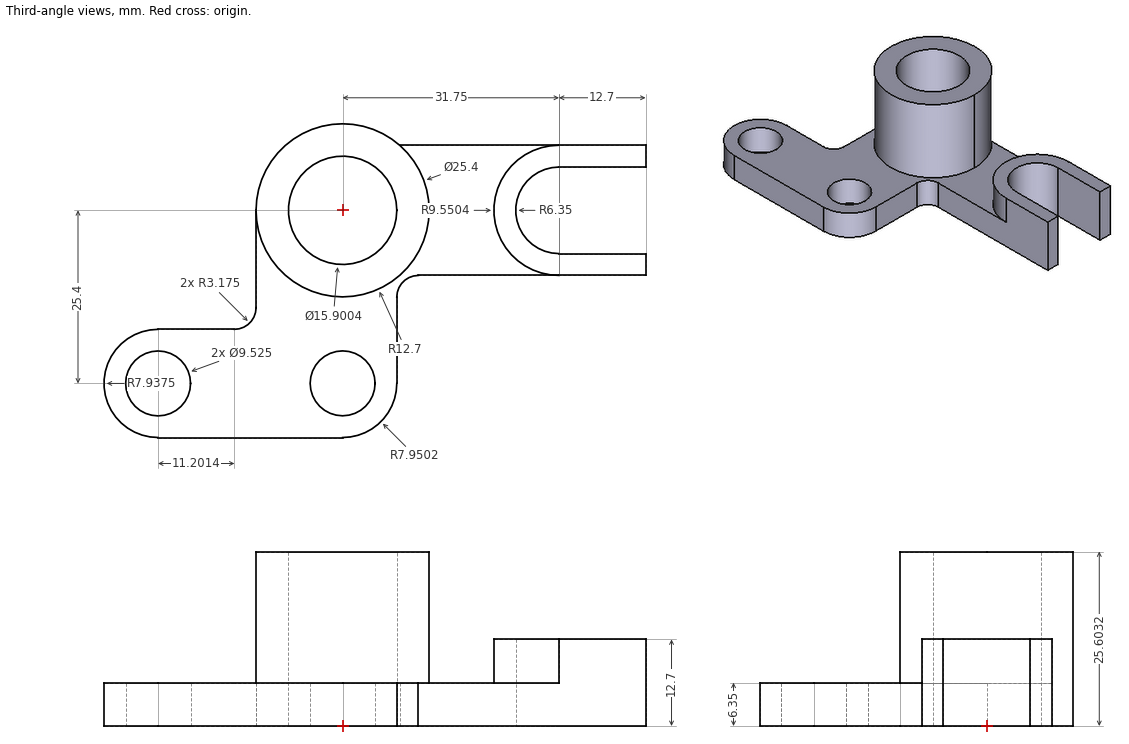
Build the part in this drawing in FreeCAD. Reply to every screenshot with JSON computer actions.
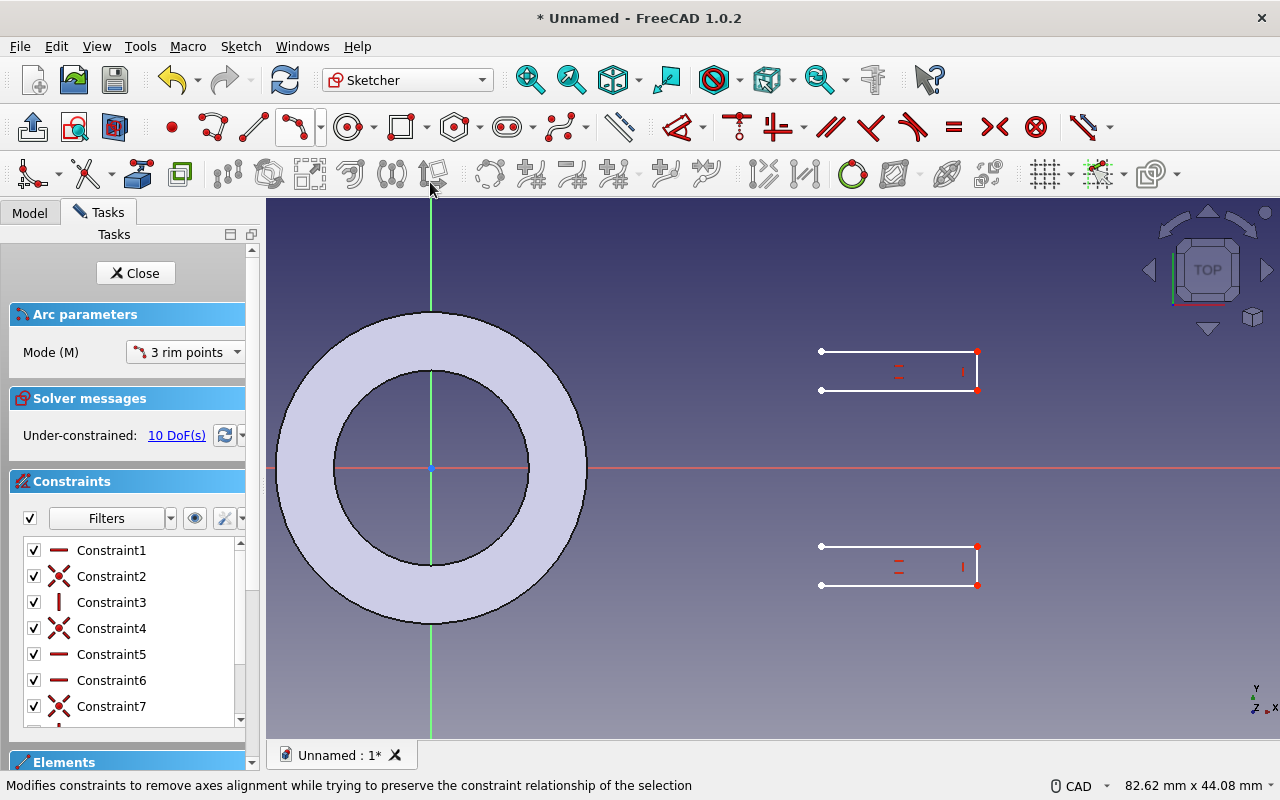
{"action": "left_click", "coordinate": [821, 547]}
{"action": "left_click", "coordinate": [821, 391]}
{"action": "left_click", "coordinate": [747, 444]}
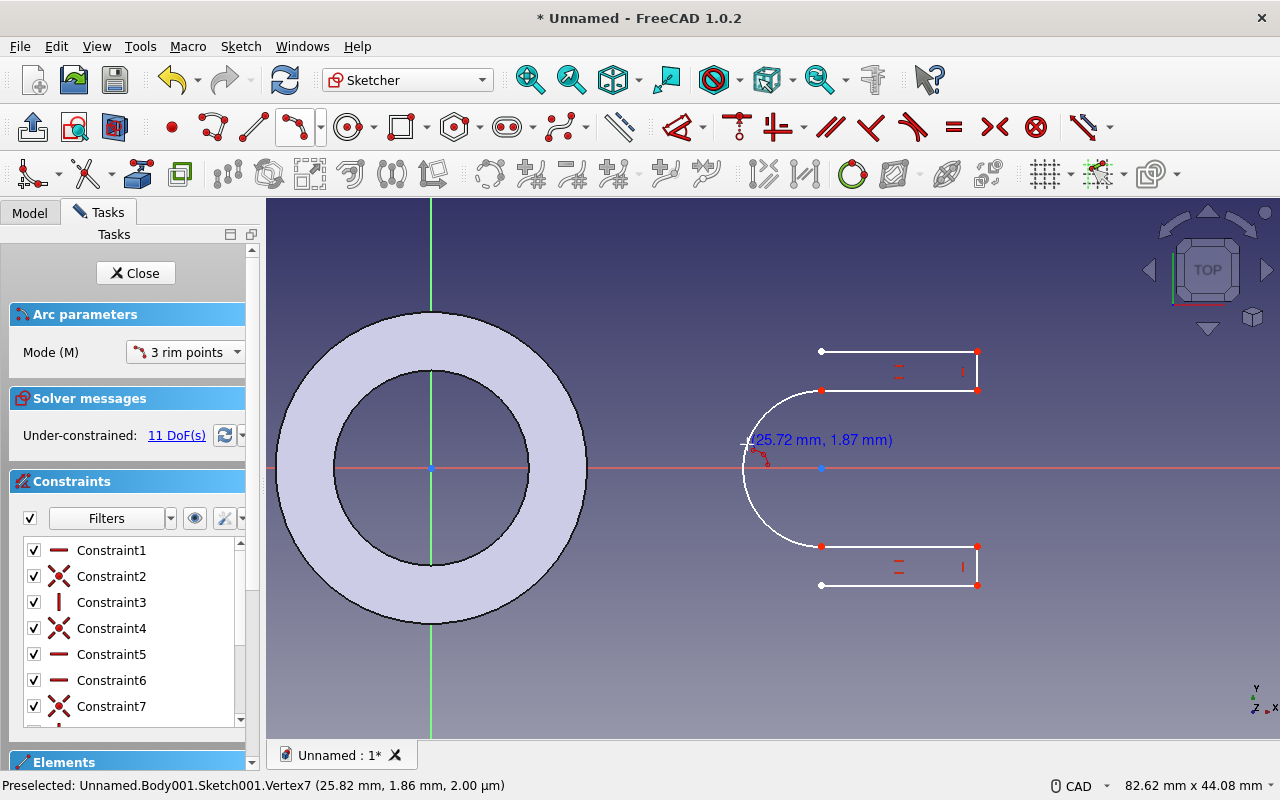
{"action": "left_click", "coordinate": [821, 352]}
{"action": "left_click", "coordinate": [821, 586]}
{"action": "left_click", "coordinate": [710, 432]}
{"action": "key", "text": "Escape"}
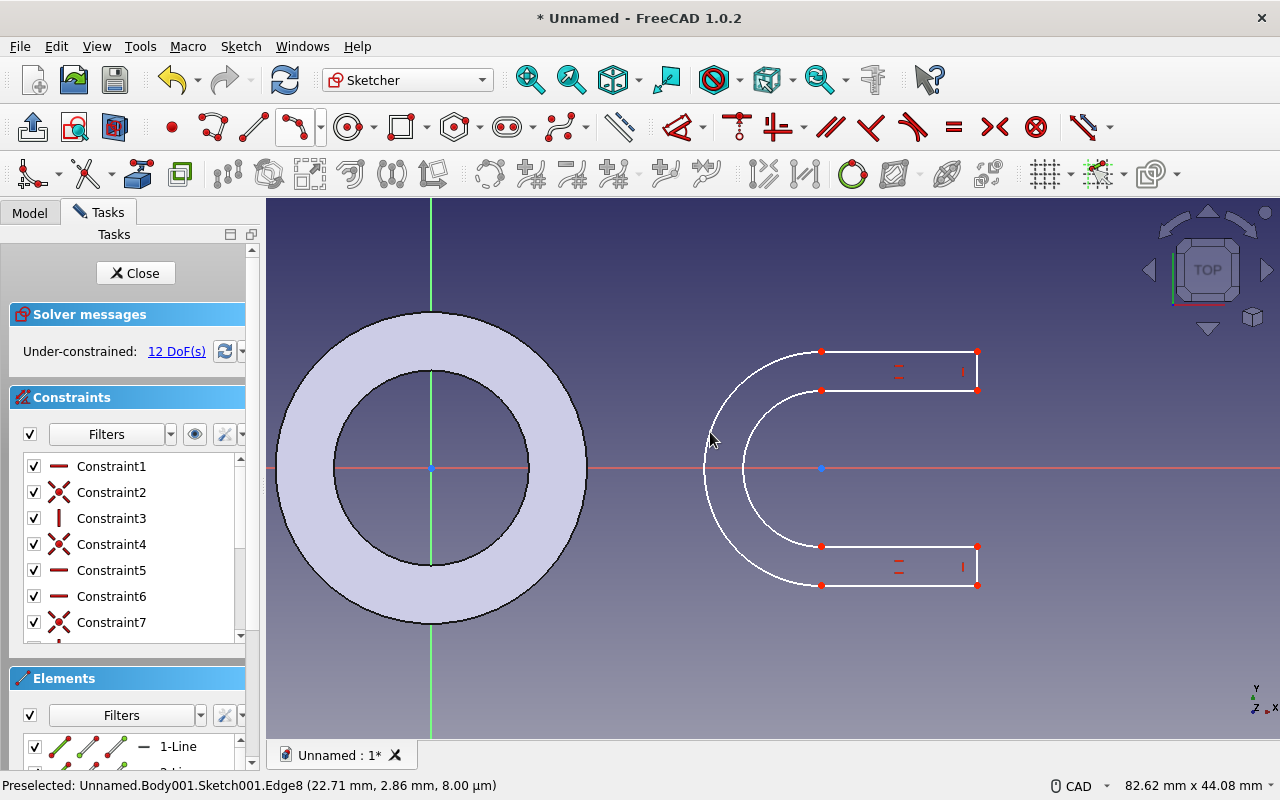
{"action": "left_click", "coordinate": [868, 586]}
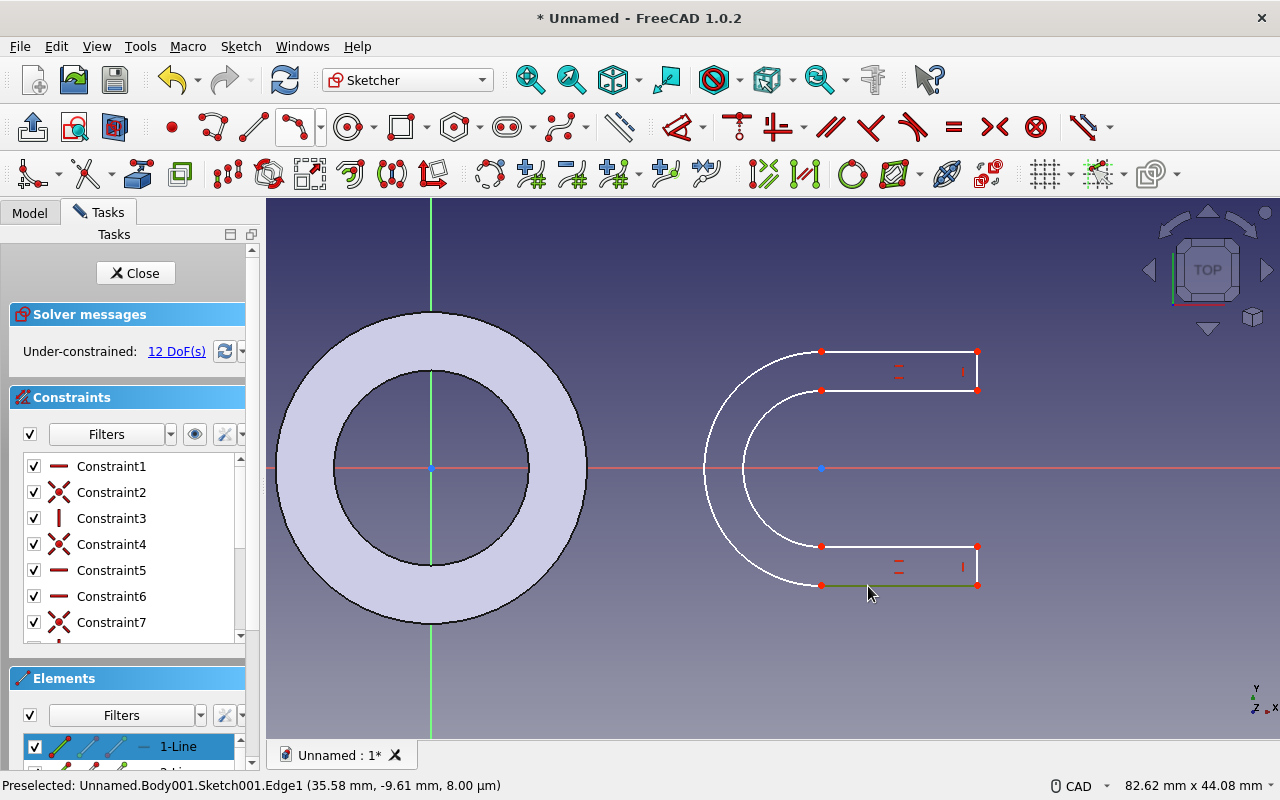
{"action": "left_click", "coordinate": [727, 400]}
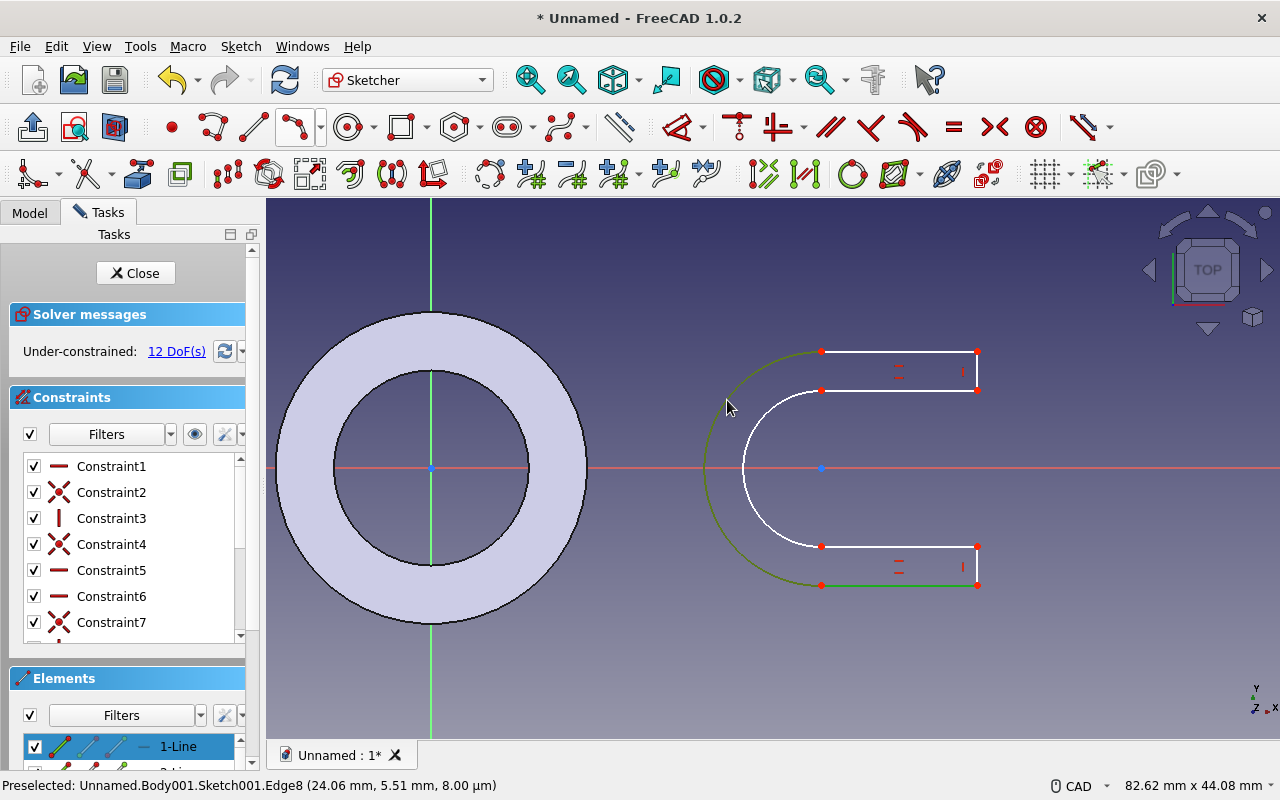
{"action": "left_click", "coordinate": [913, 128]}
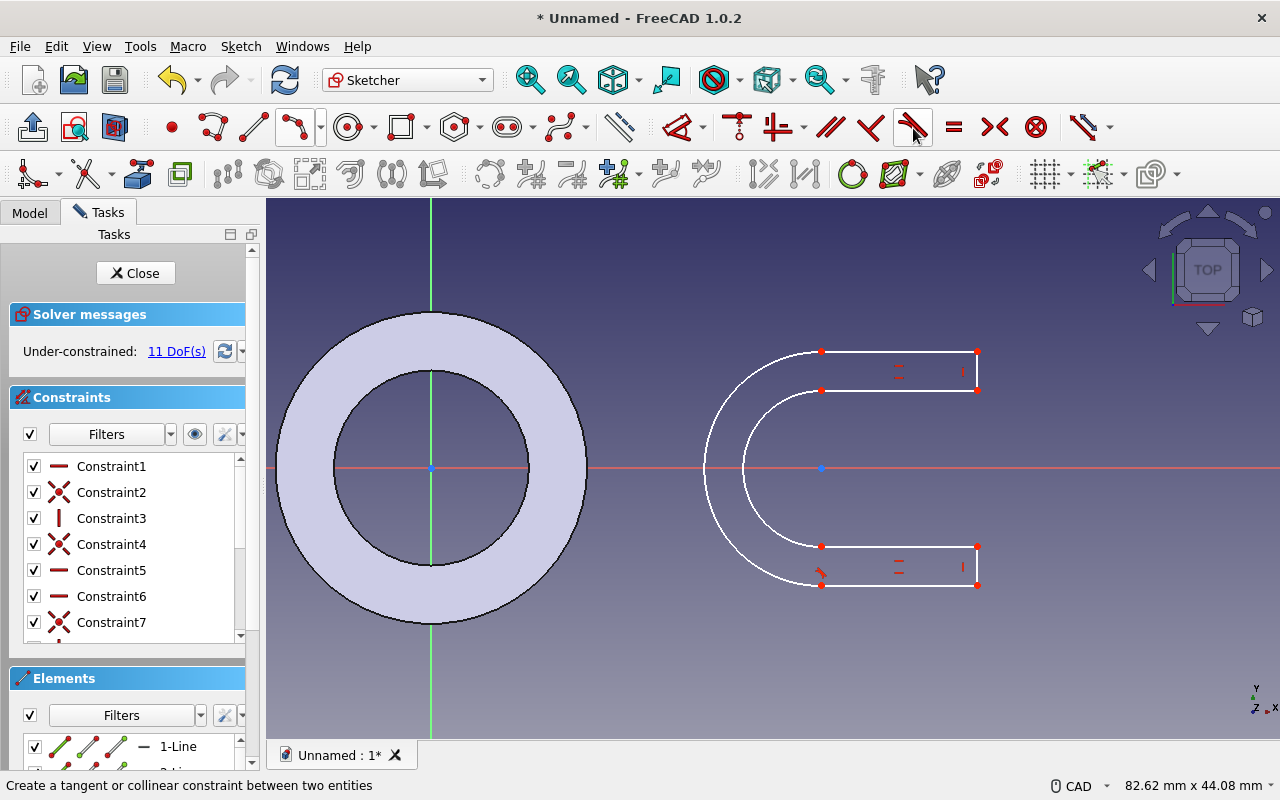
{"action": "left_click", "coordinate": [930, 547]}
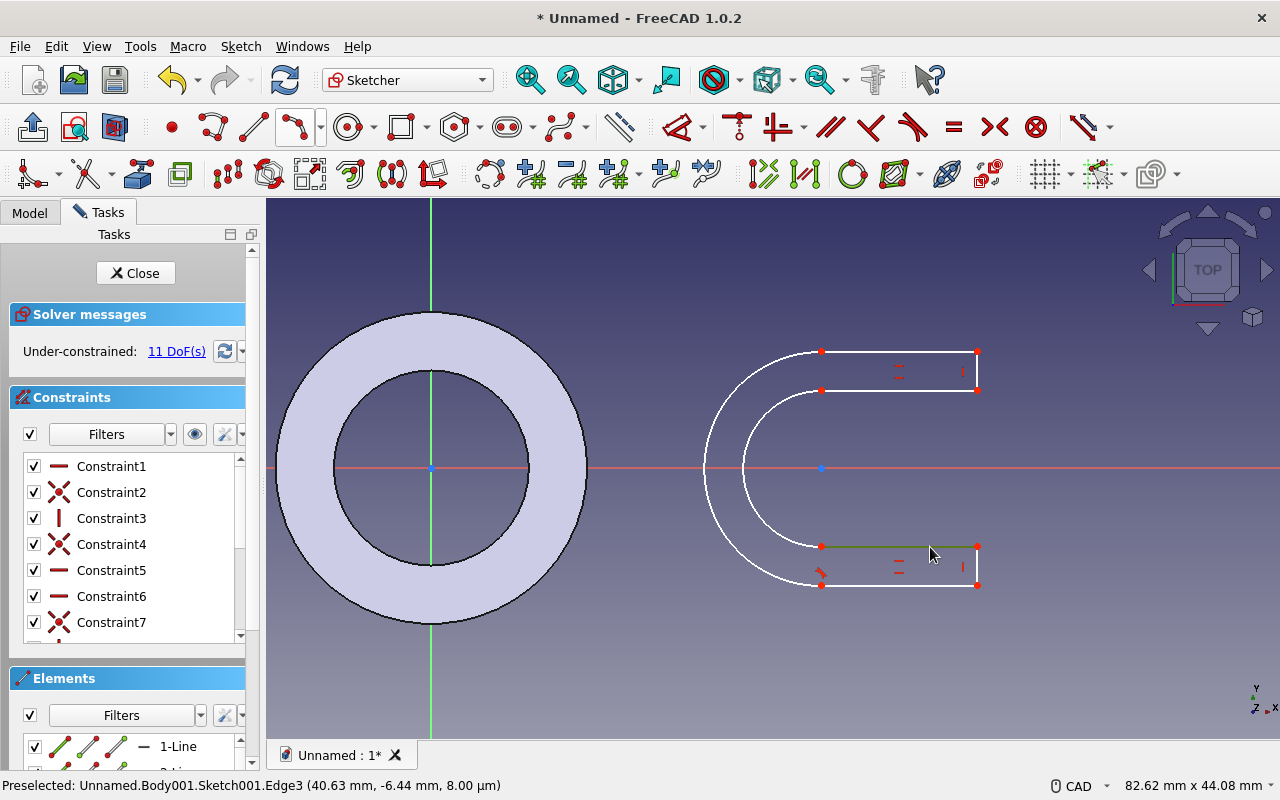
{"action": "left_click", "coordinate": [758, 423]}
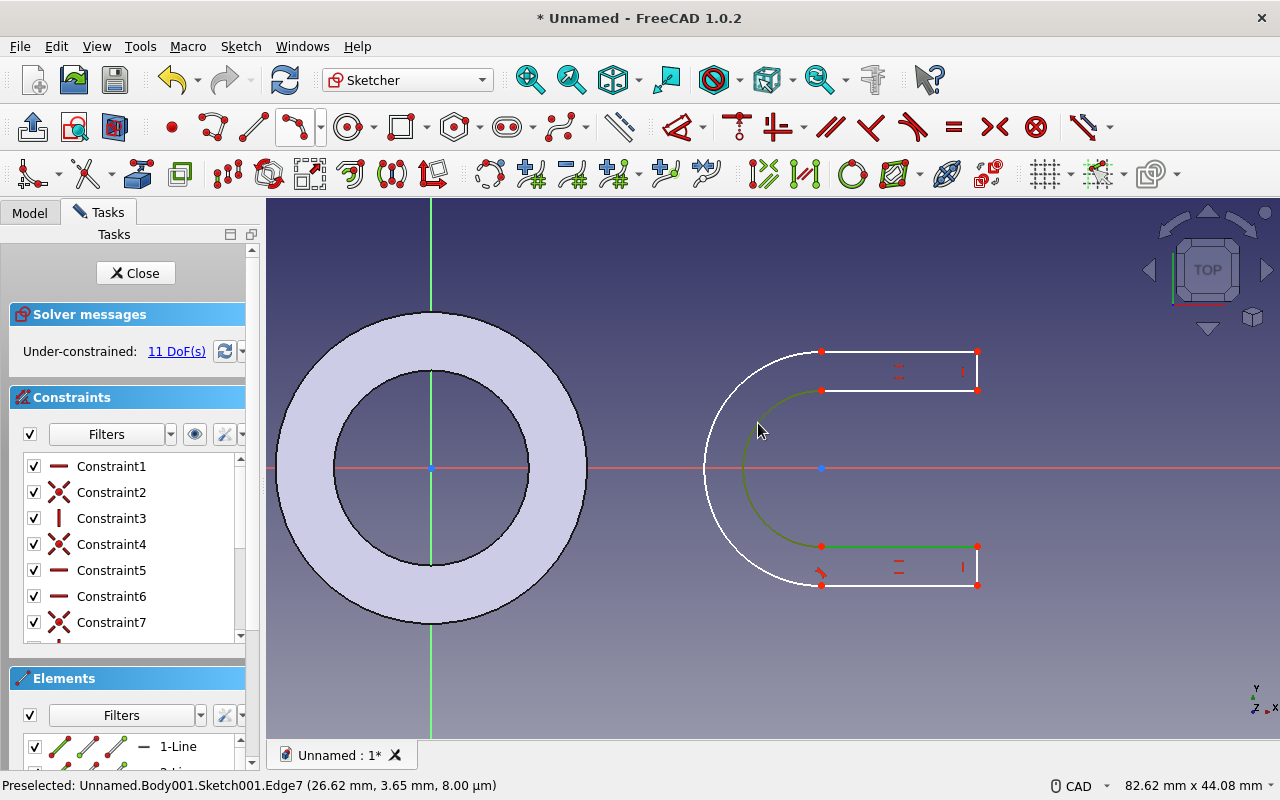
{"action": "key", "text": "t"}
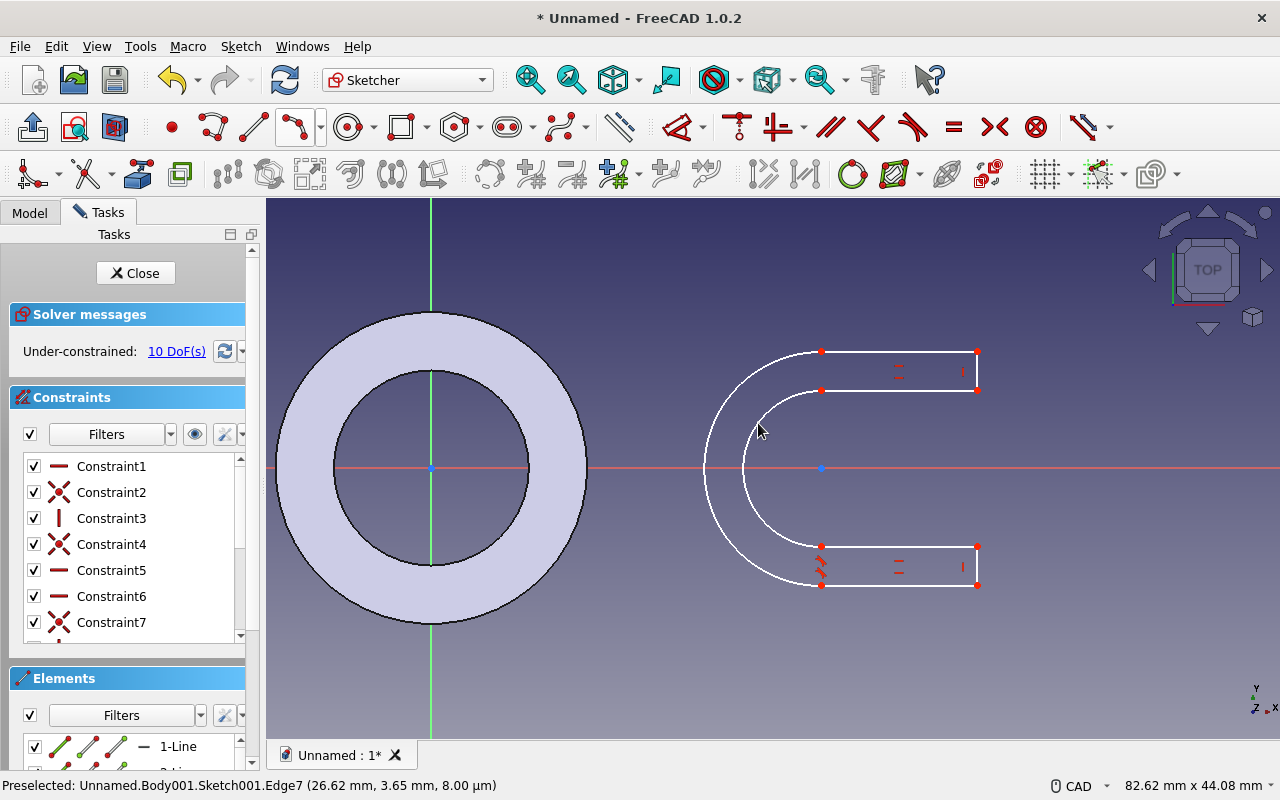
{"action": "left_click", "coordinate": [868, 391]}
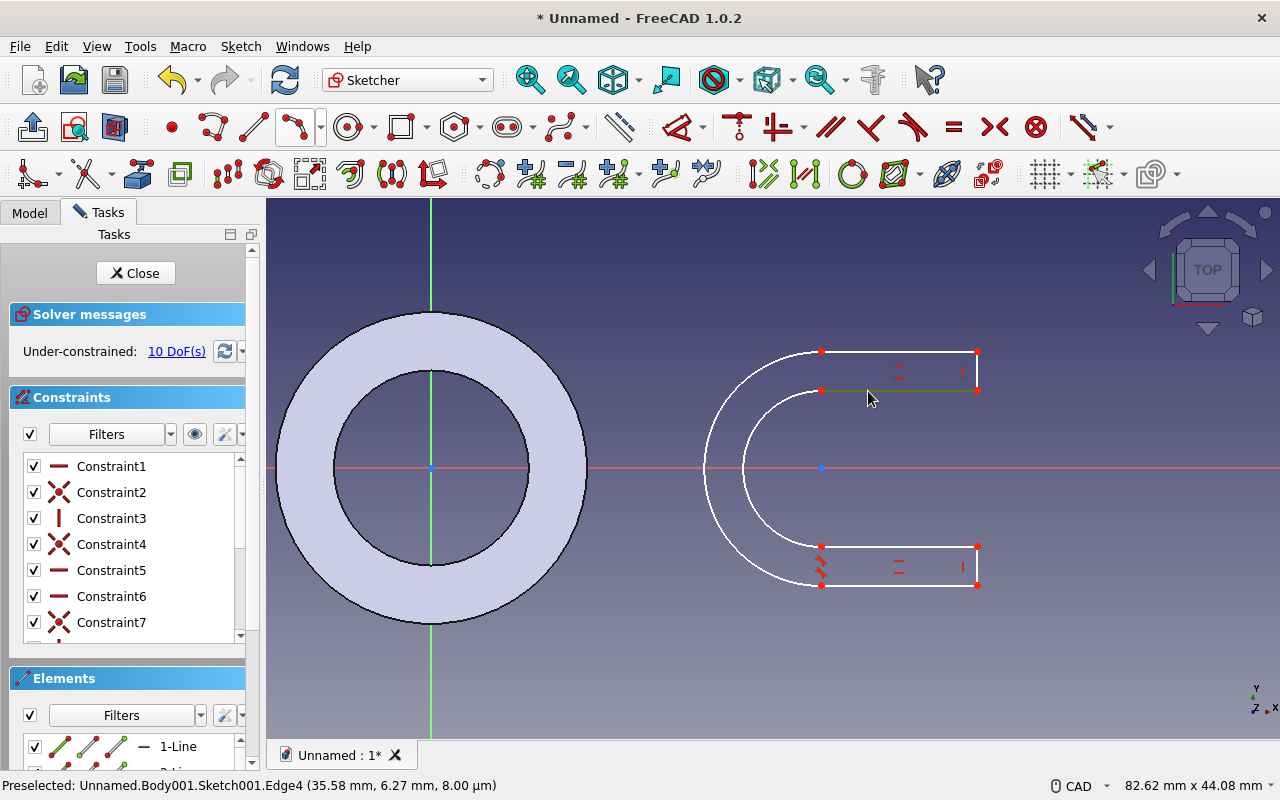
{"action": "left_click", "coordinate": [758, 423]}